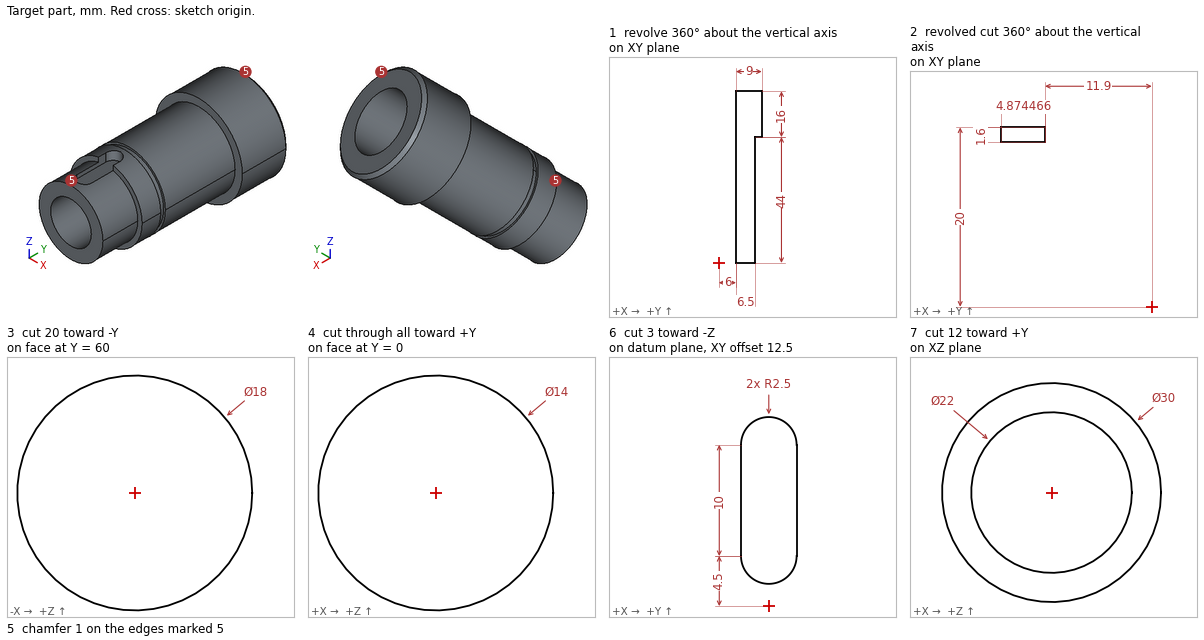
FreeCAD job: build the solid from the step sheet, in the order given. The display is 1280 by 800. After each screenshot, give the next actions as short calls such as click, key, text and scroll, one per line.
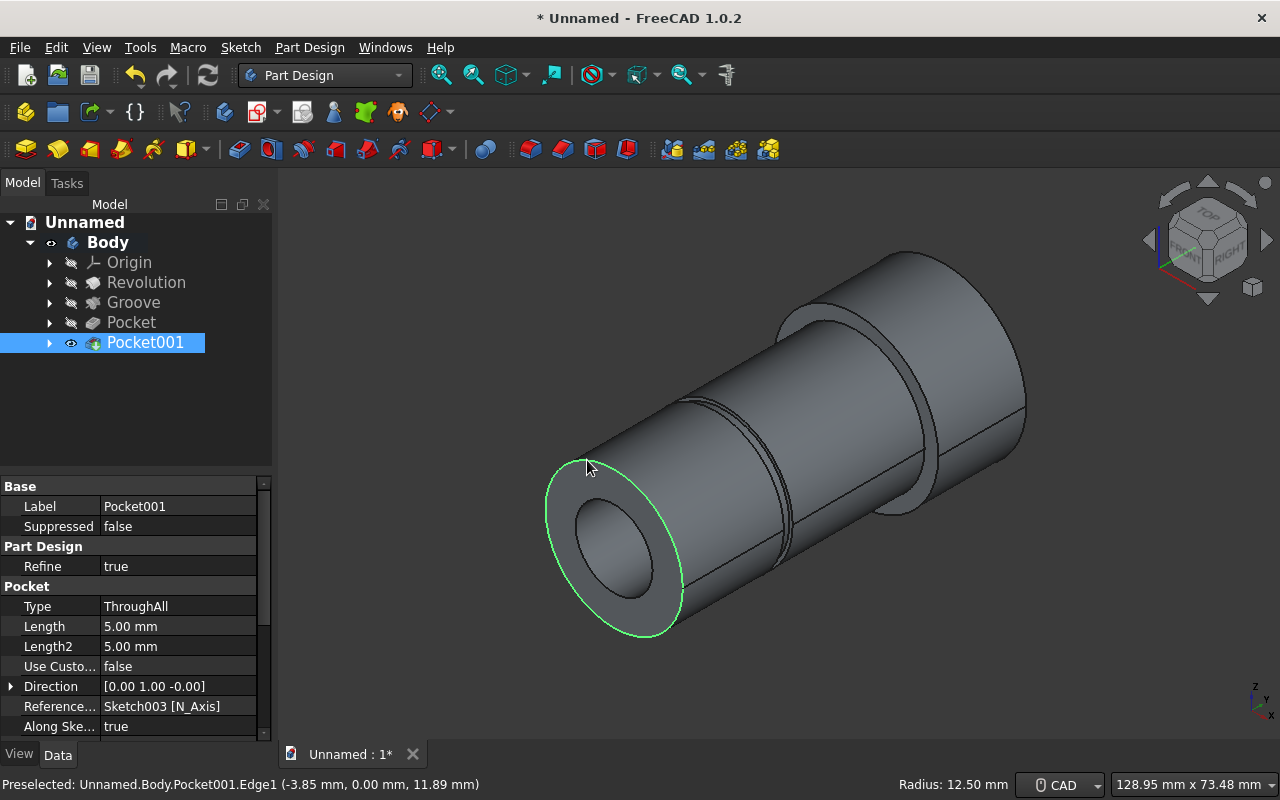
click(918, 252, ctrl)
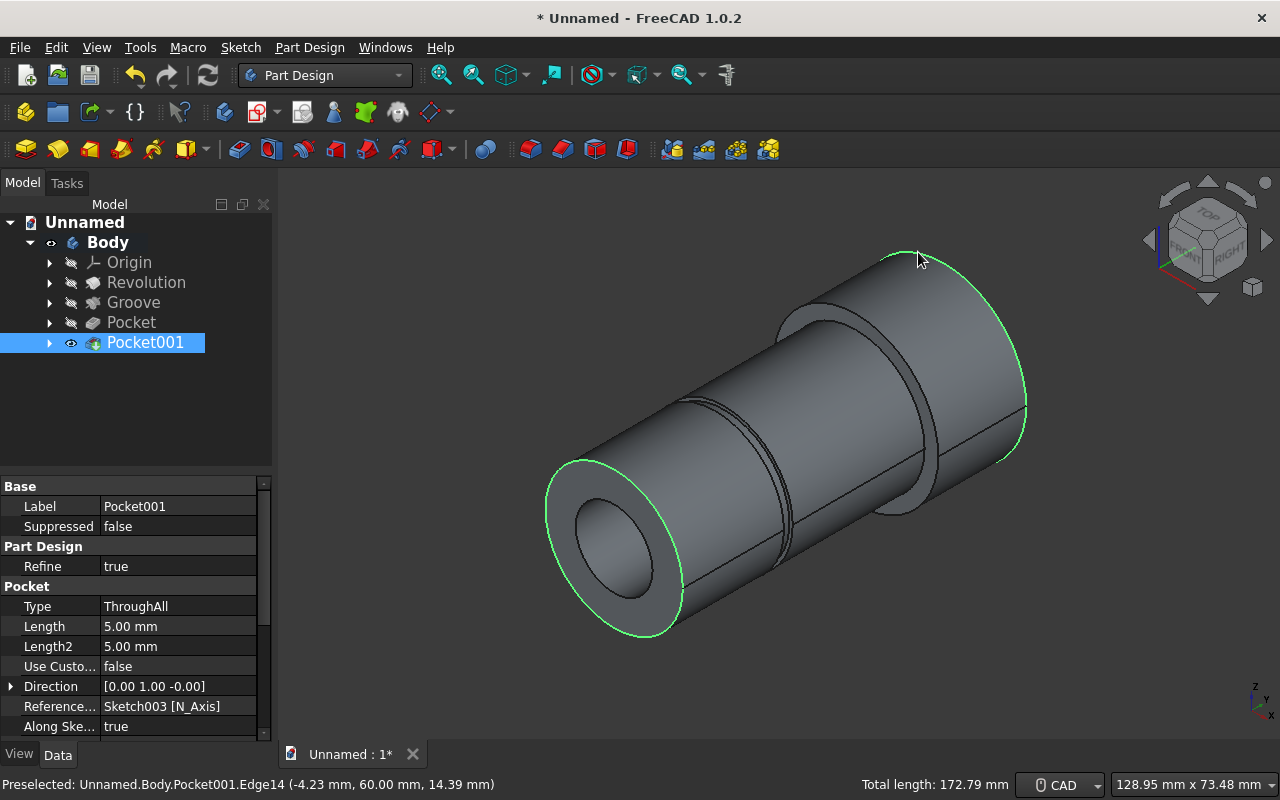
click(564, 150)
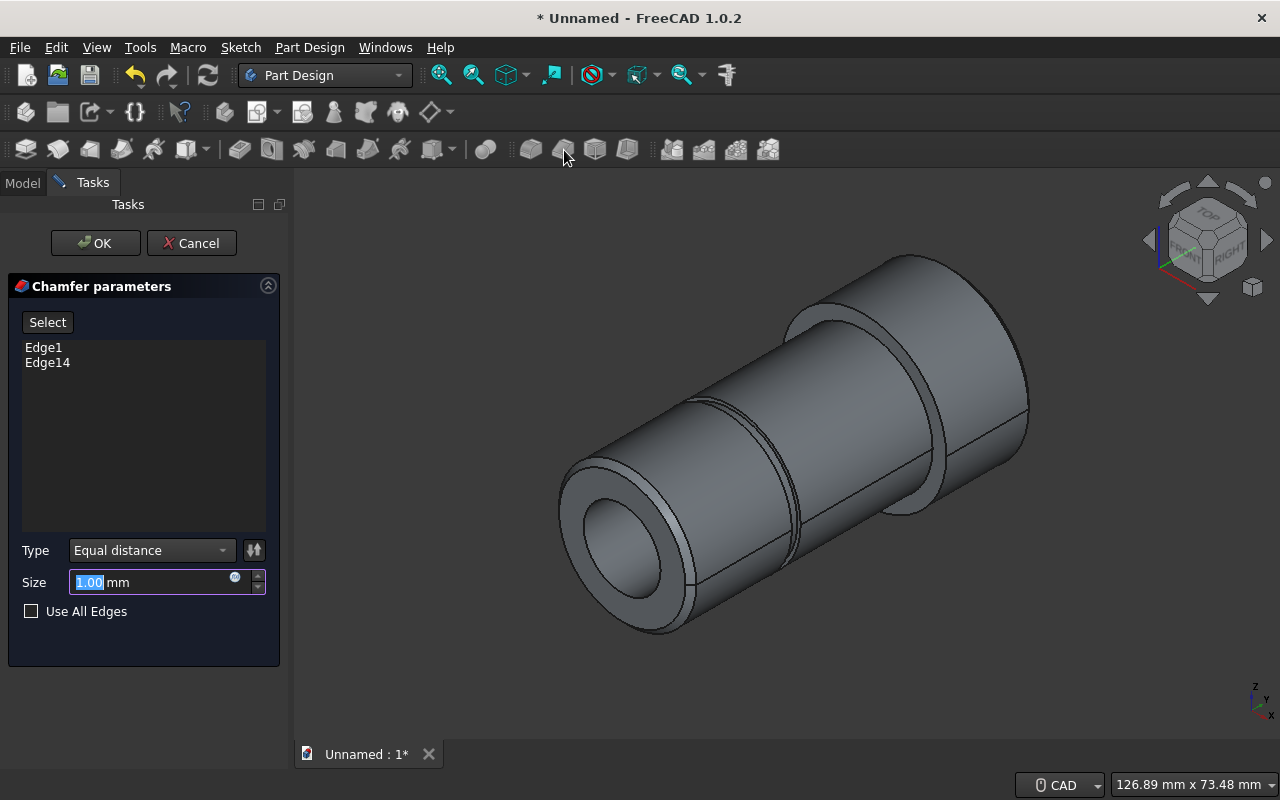
text(1)
key(Tab)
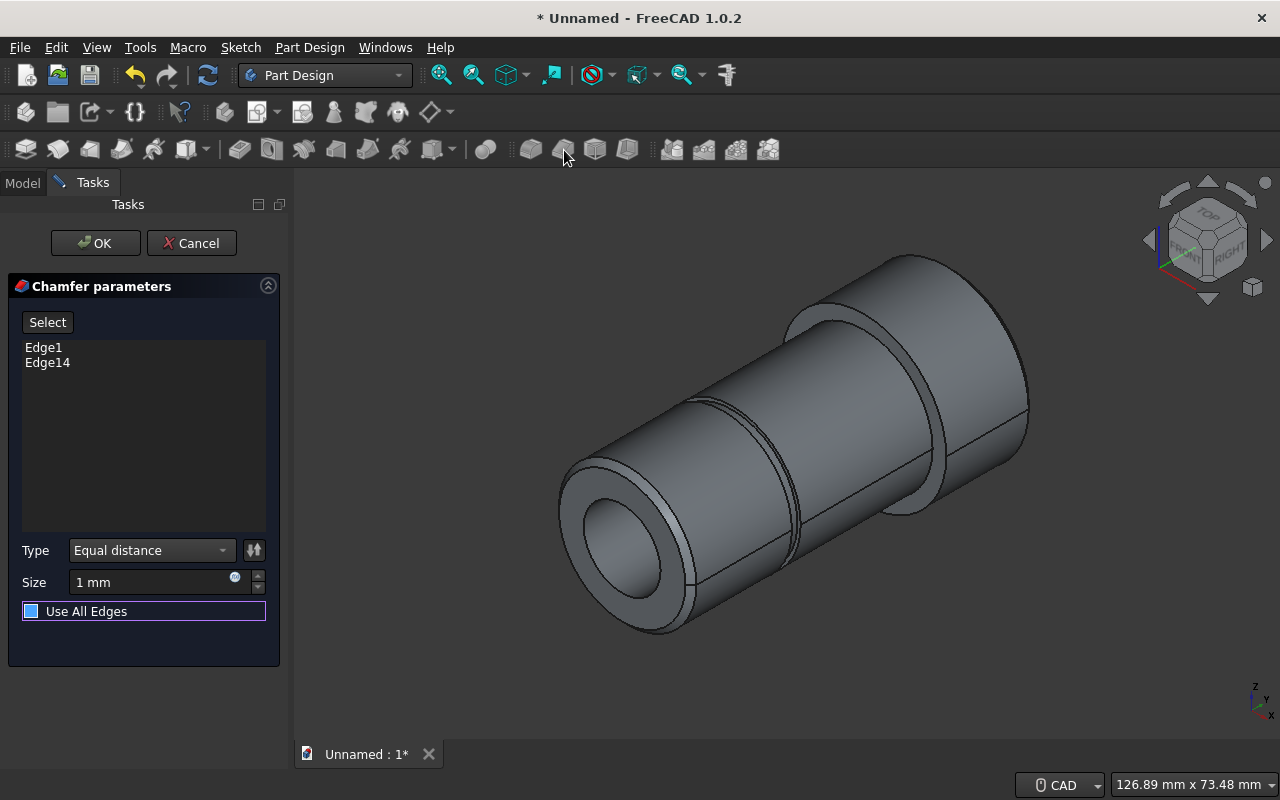
click(96, 243)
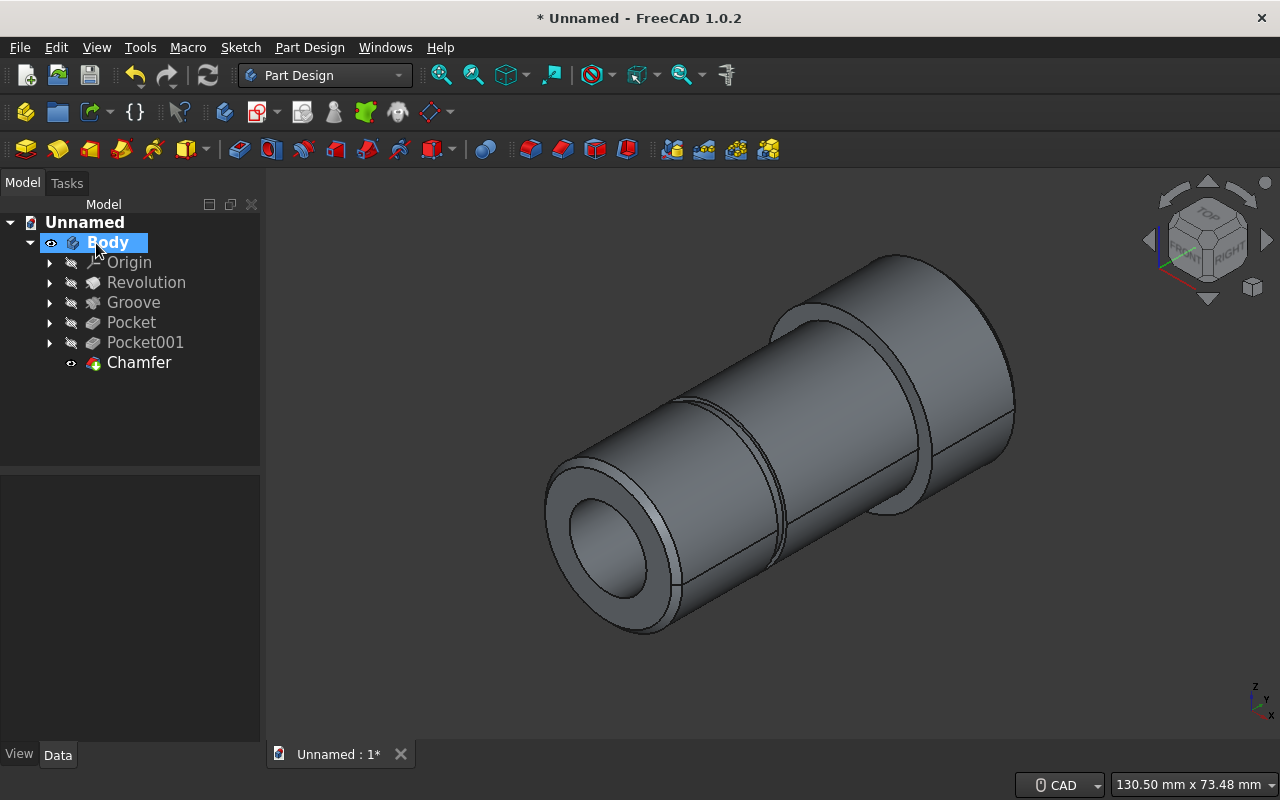
click(50, 263)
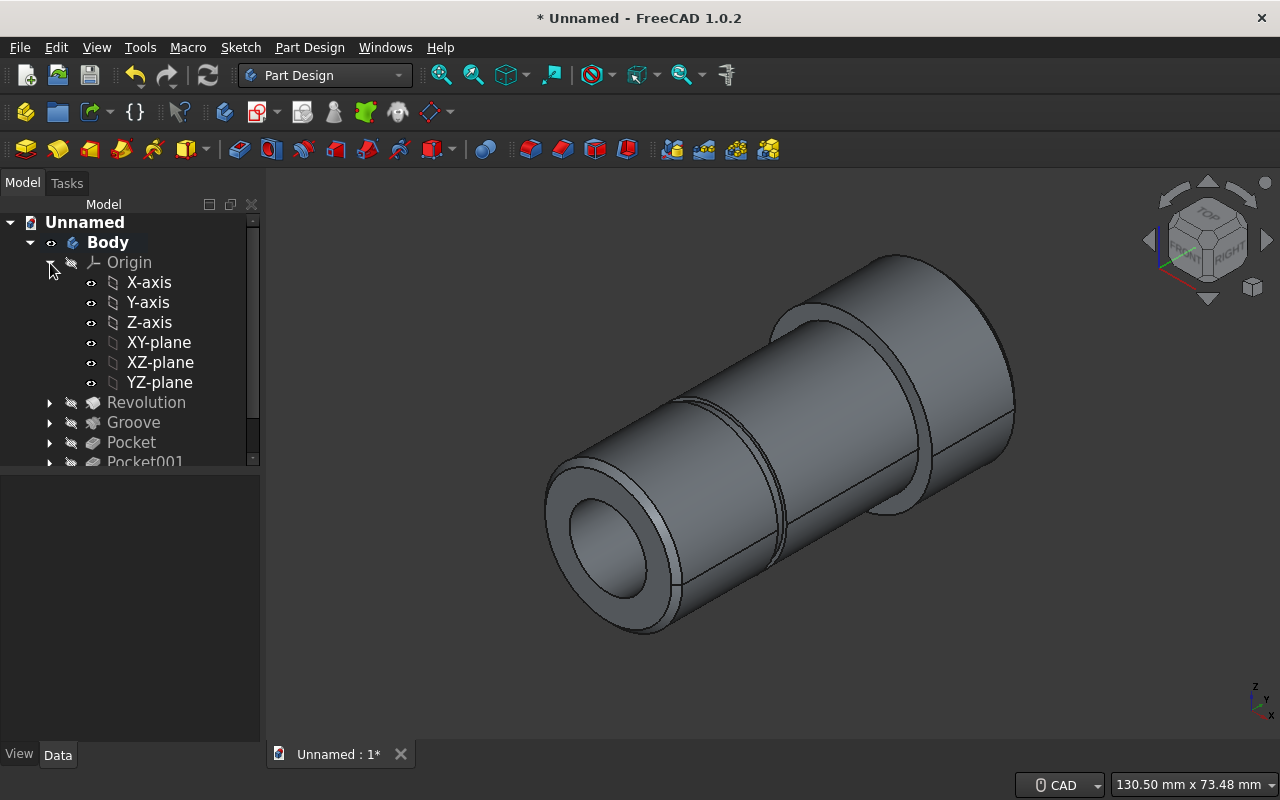
click(136, 343)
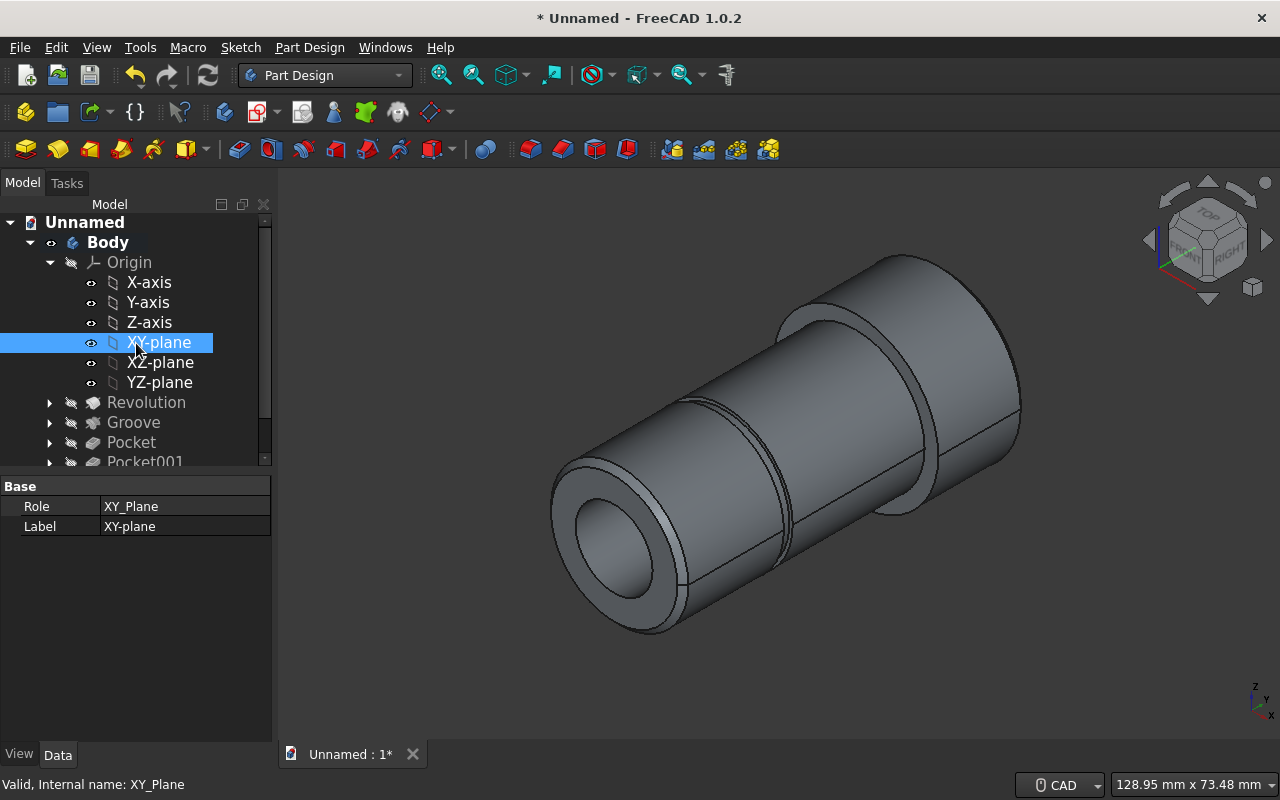
click(430, 112)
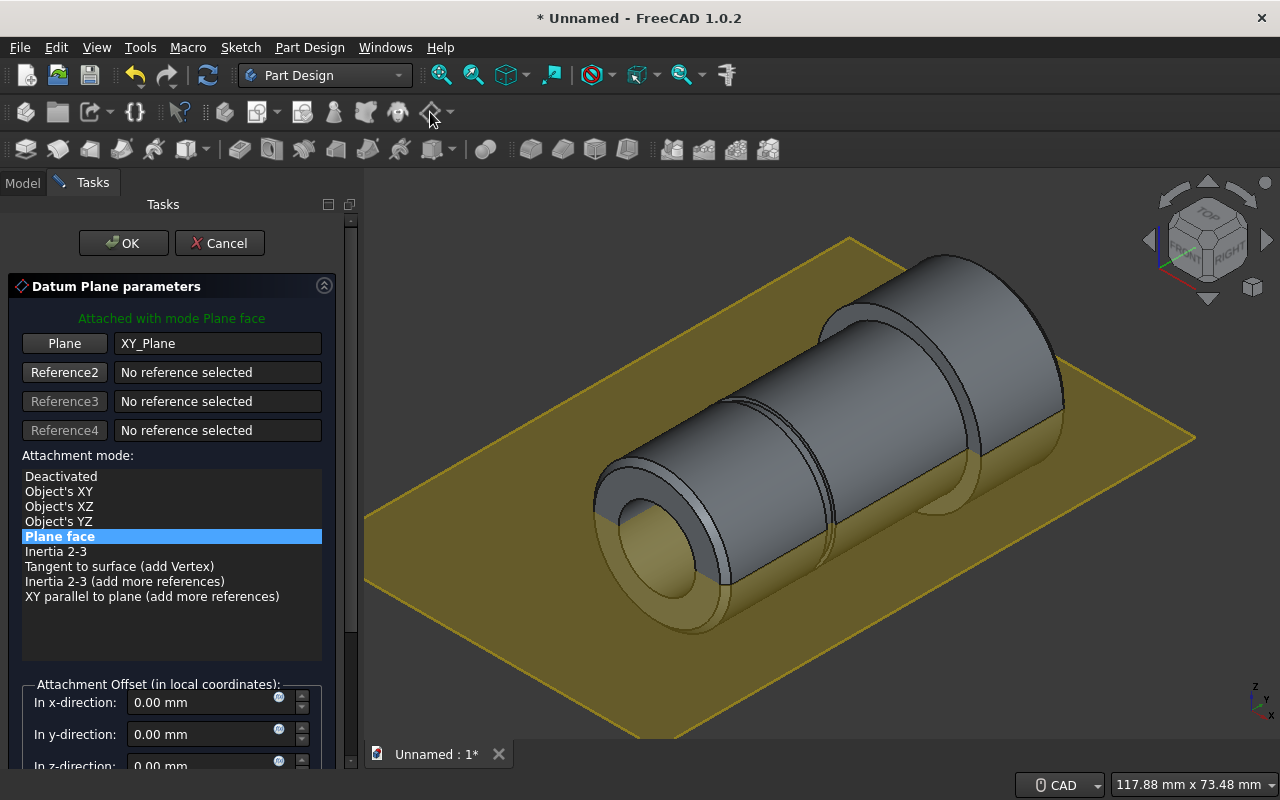
scroll(351, 491, down, 2)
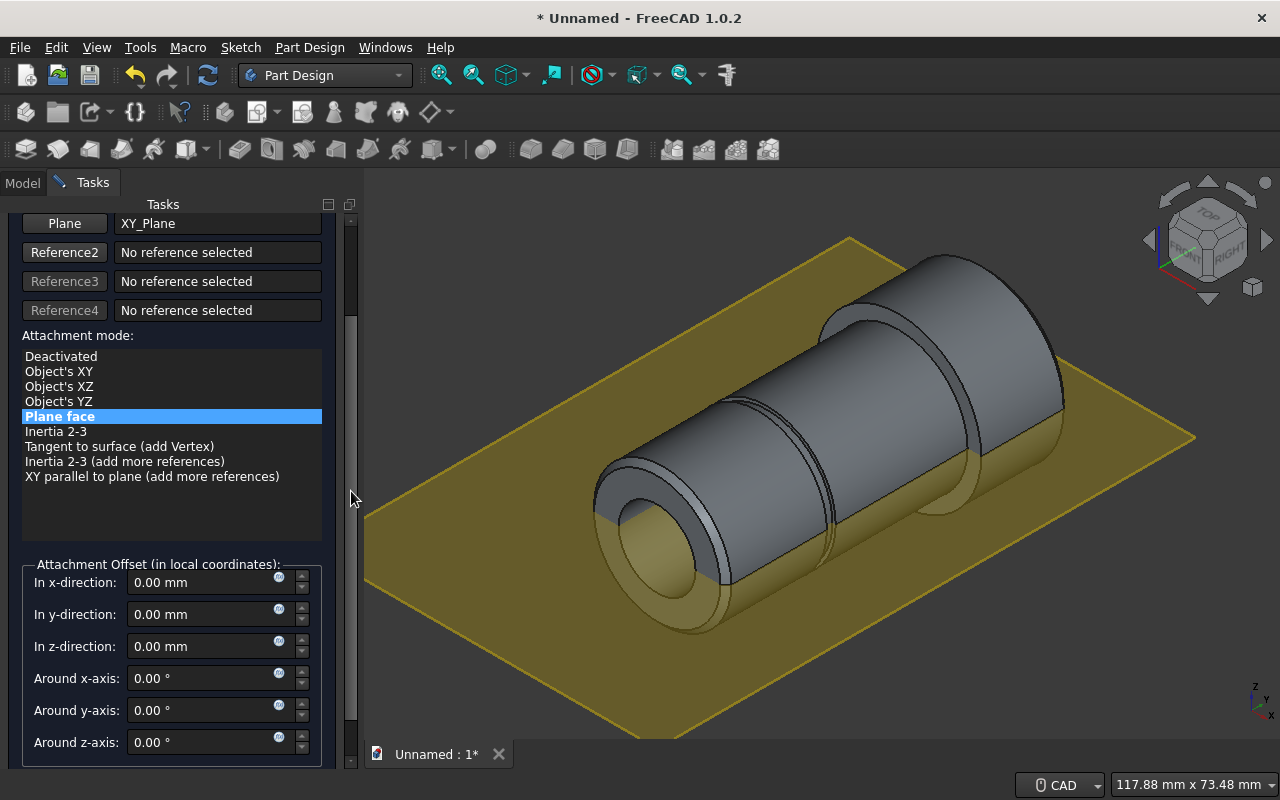
triple_click(210, 646)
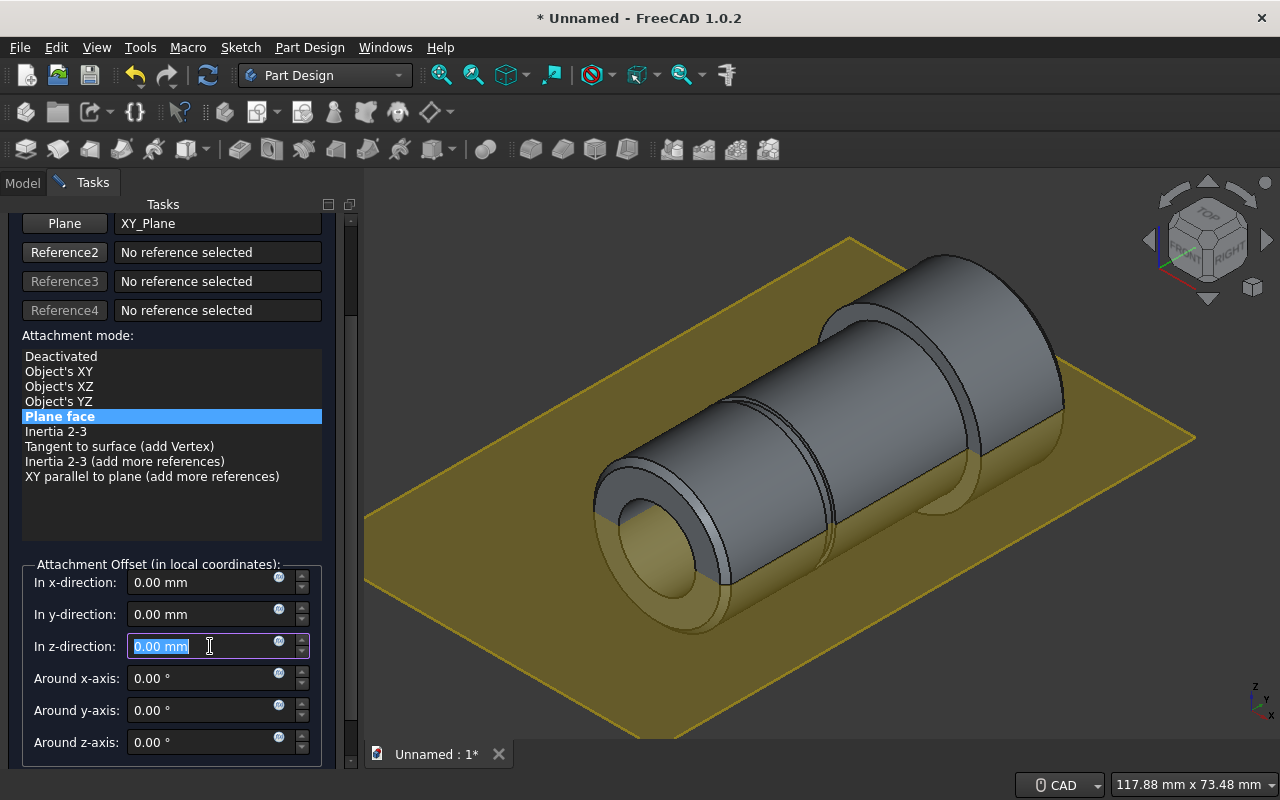
text(12.5)
key(Tab)